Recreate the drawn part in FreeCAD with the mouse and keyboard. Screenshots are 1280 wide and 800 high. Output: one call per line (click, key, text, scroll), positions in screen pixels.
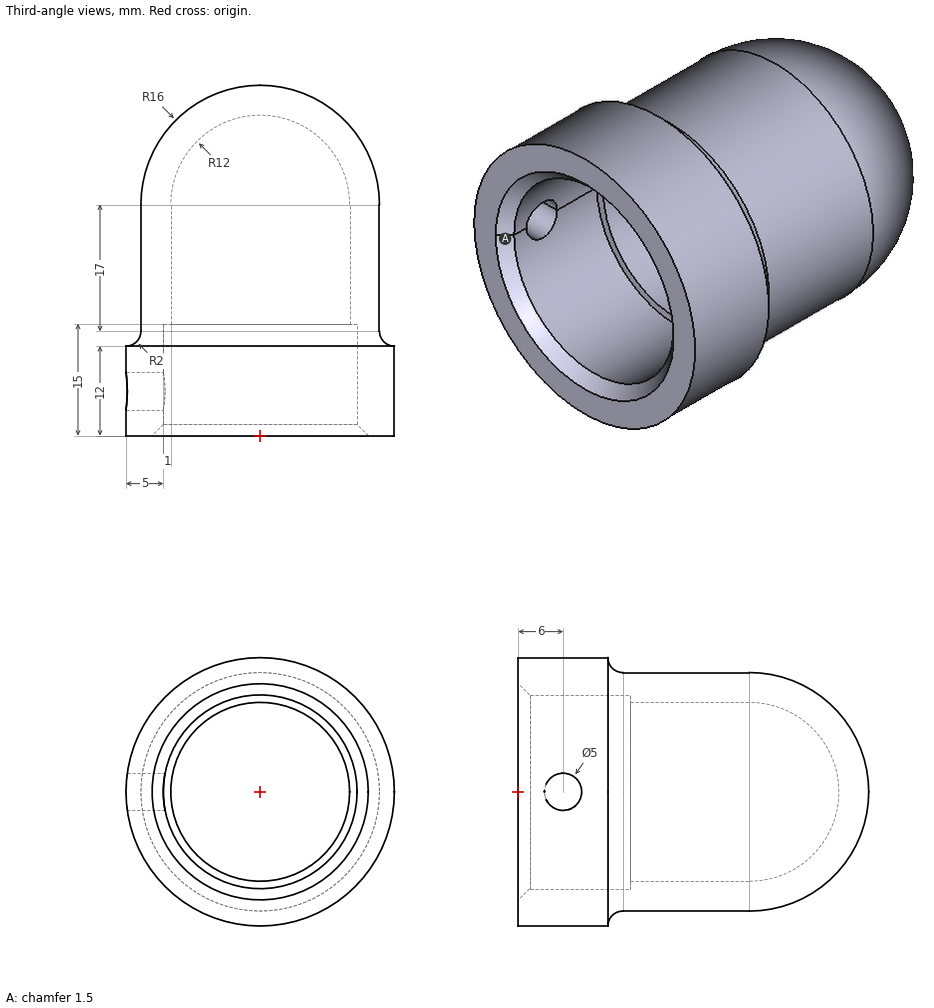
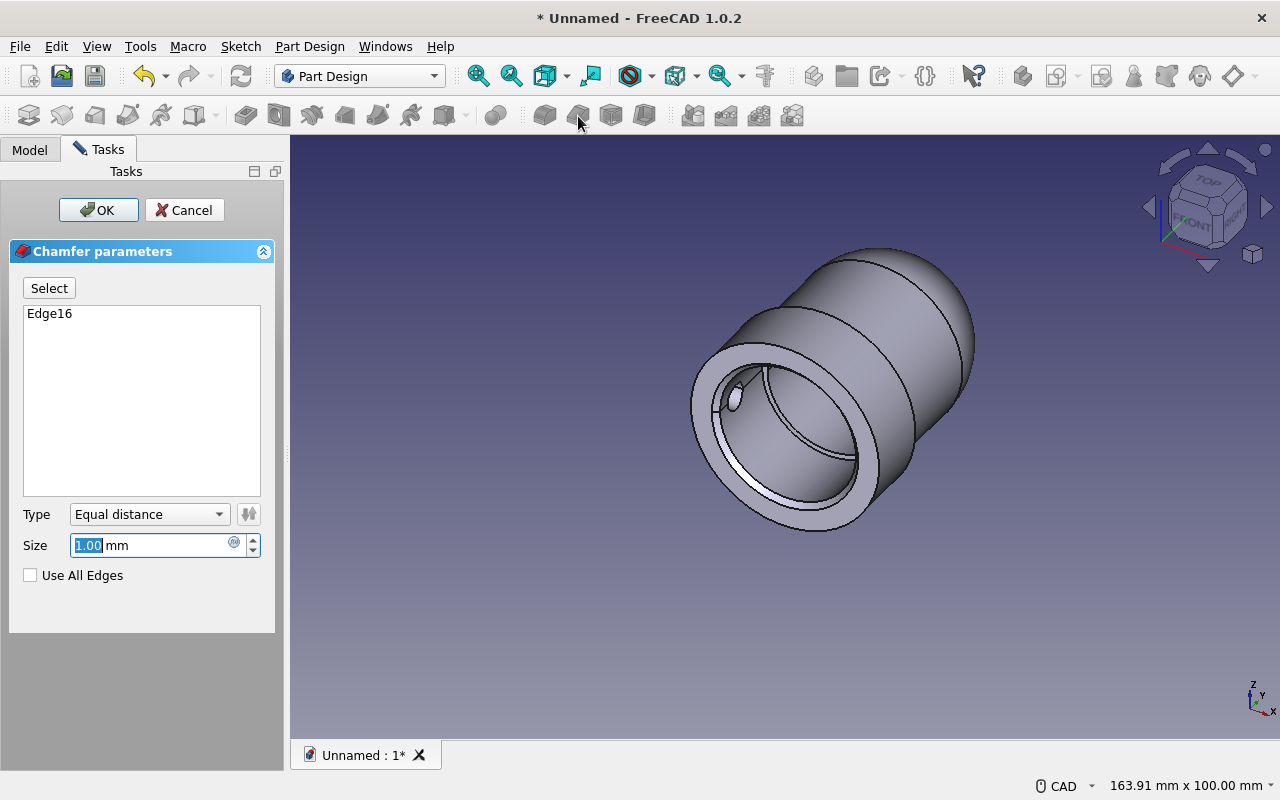
text(1.5)
key(Tab)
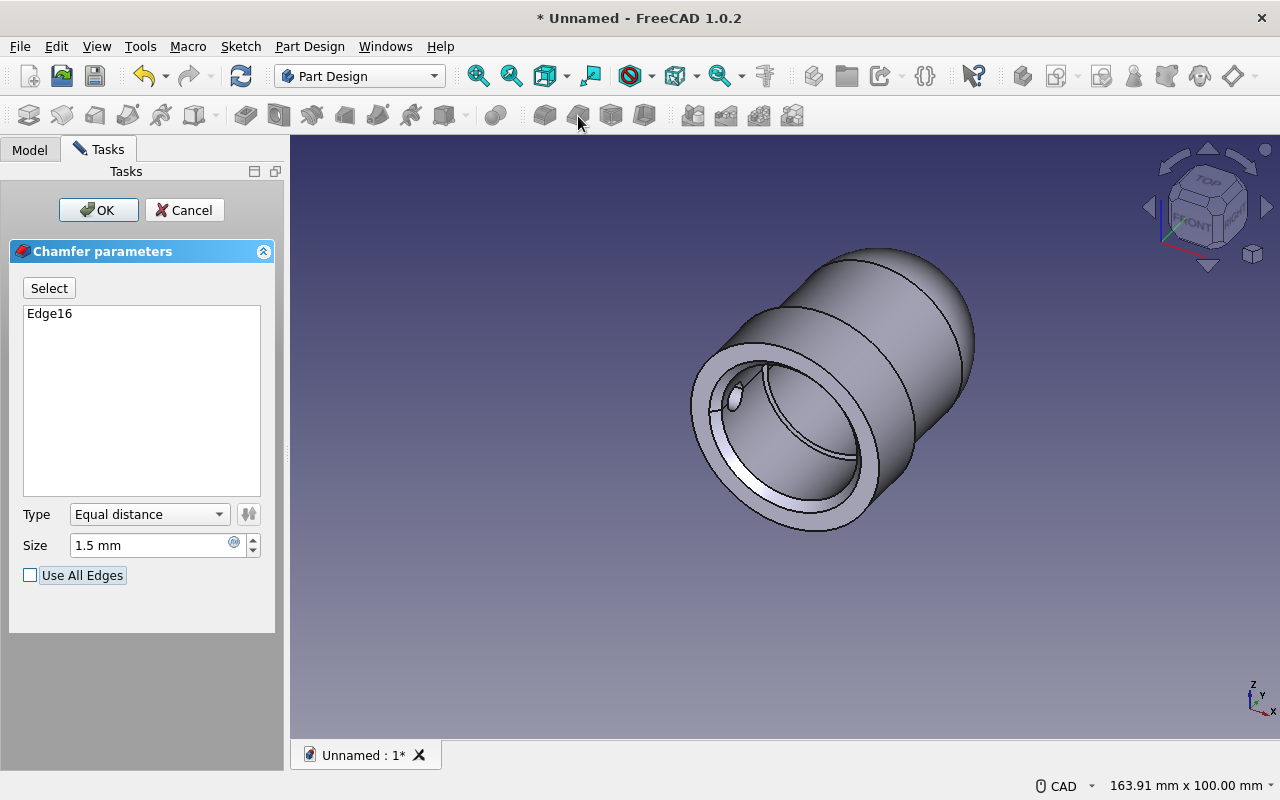
click(99, 210)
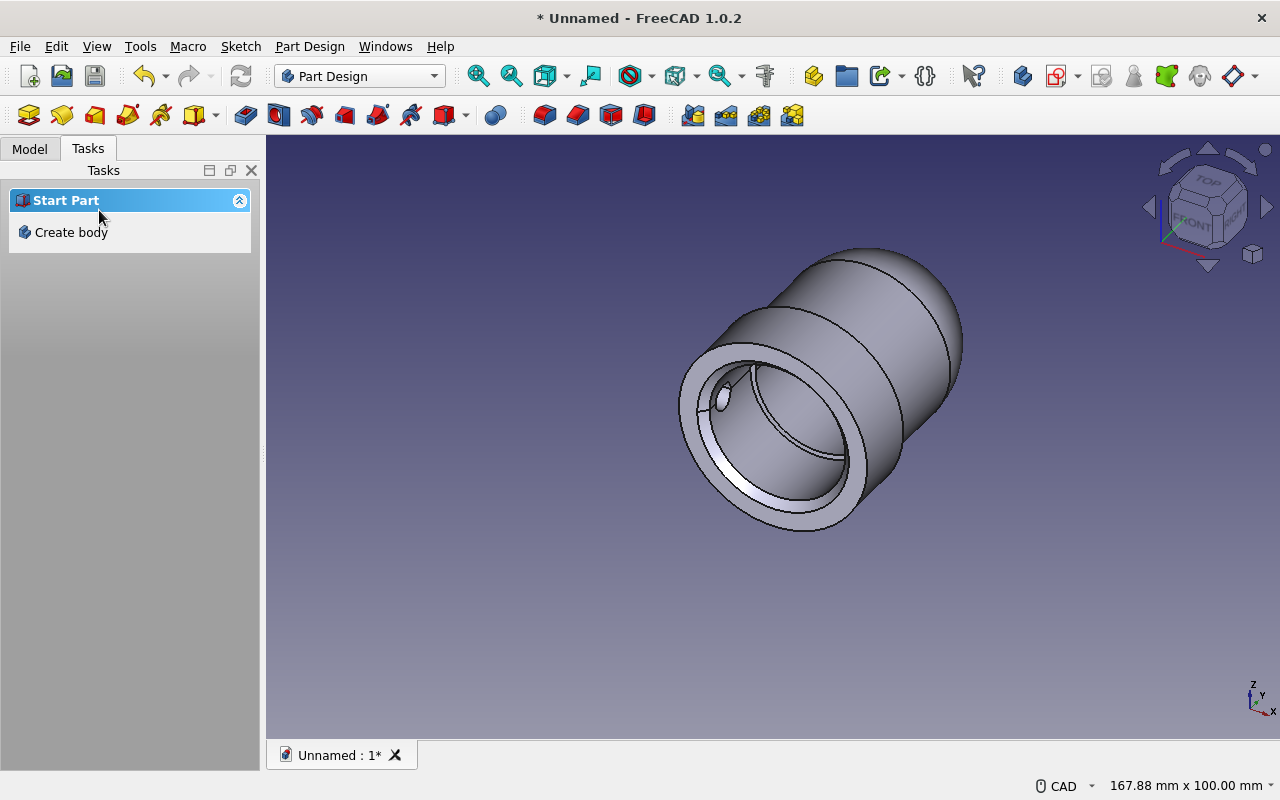
key(0)